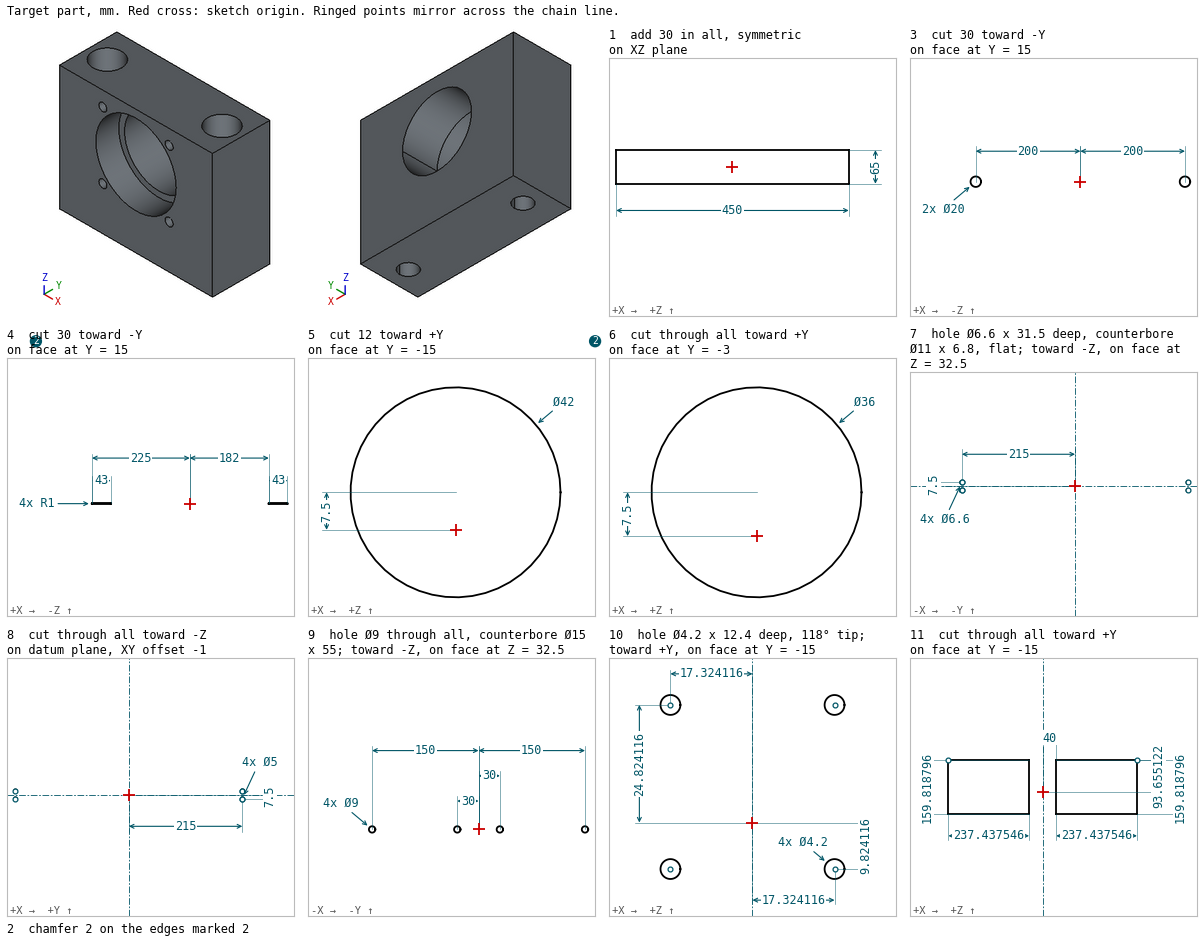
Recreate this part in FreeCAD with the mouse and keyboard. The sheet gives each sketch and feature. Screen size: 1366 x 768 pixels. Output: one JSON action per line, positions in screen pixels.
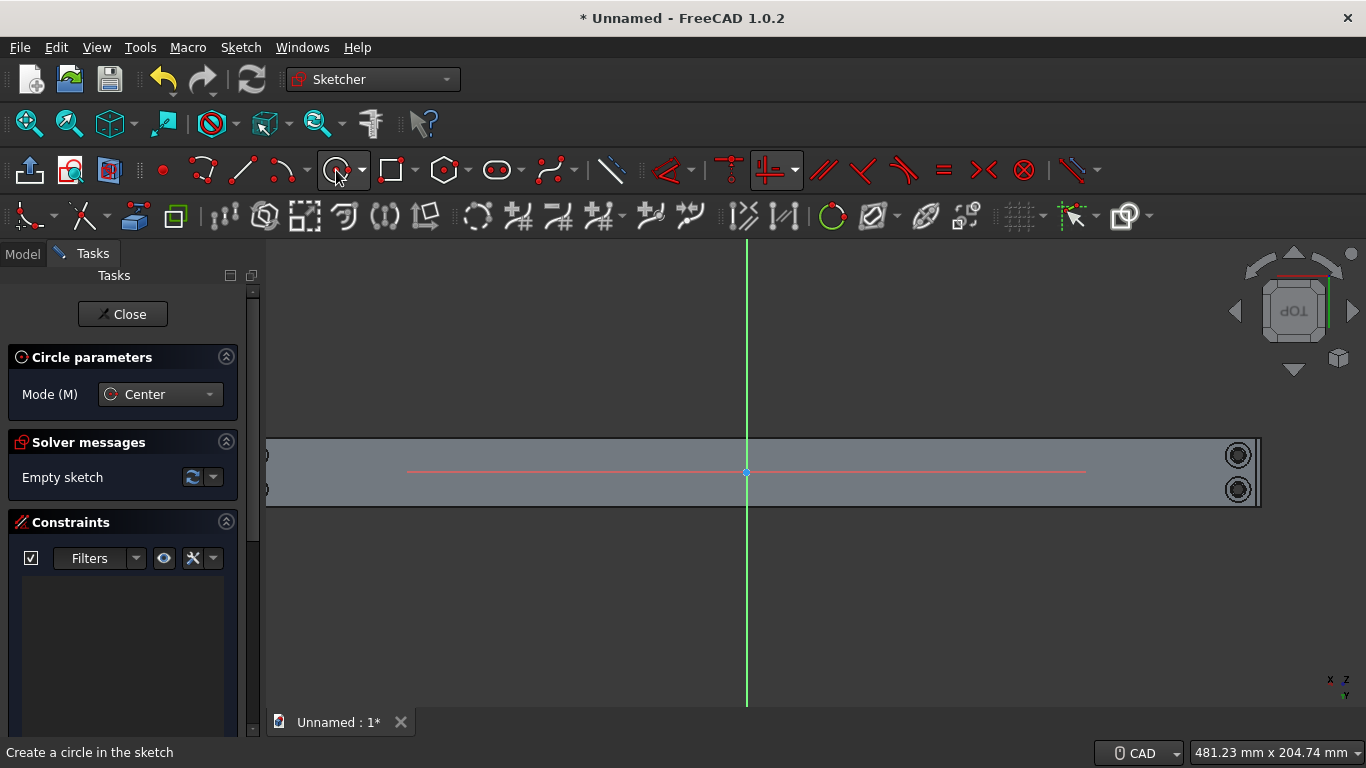
{"action": "scroll", "coordinate": [404, 472], "scroll_direction": "up", "scroll_amount": 4}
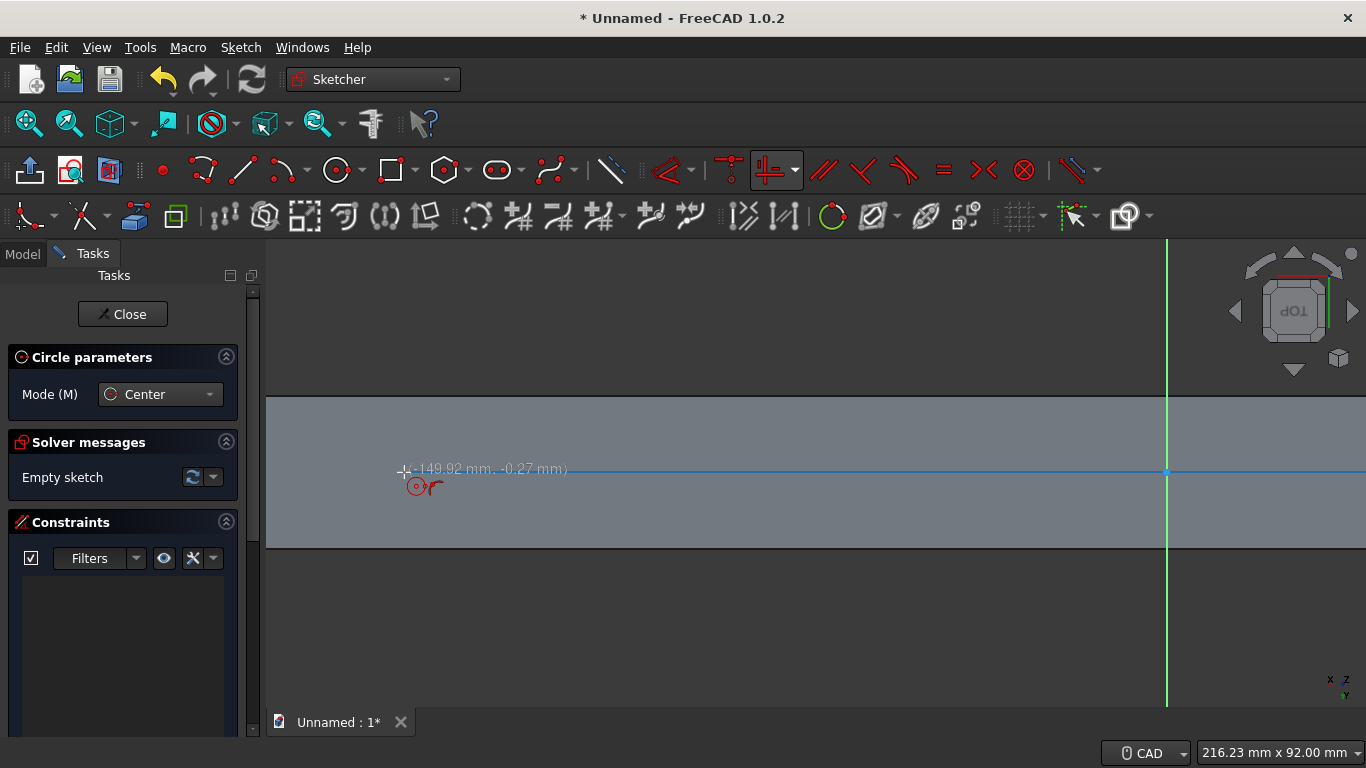
{"action": "left_click", "coordinate": [403, 472]}
{"action": "mouse_move", "coordinate": [420, 456]}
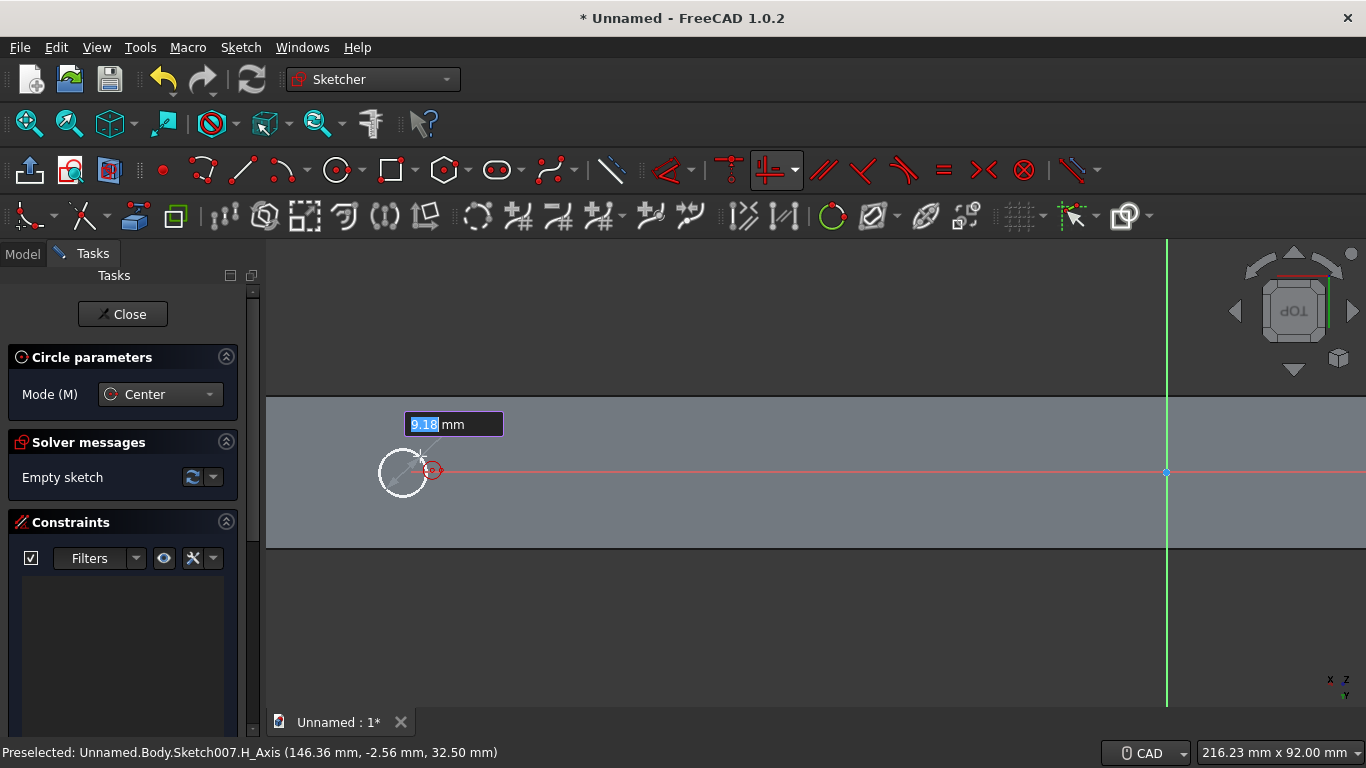
{"action": "type", "text": "9"}
{"action": "key", "text": "Return"}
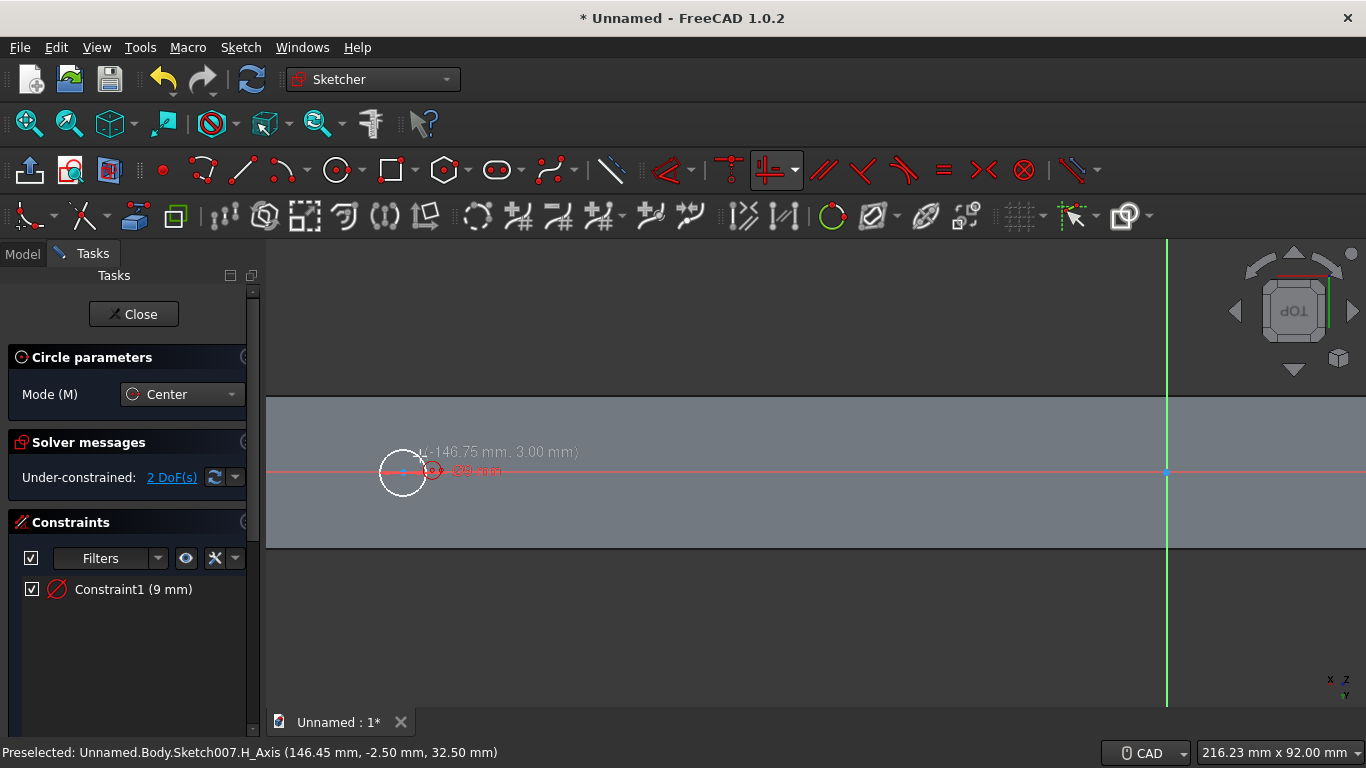
{"action": "left_click", "coordinate": [1014, 472]}
{"action": "mouse_move", "coordinate": [1030, 456]}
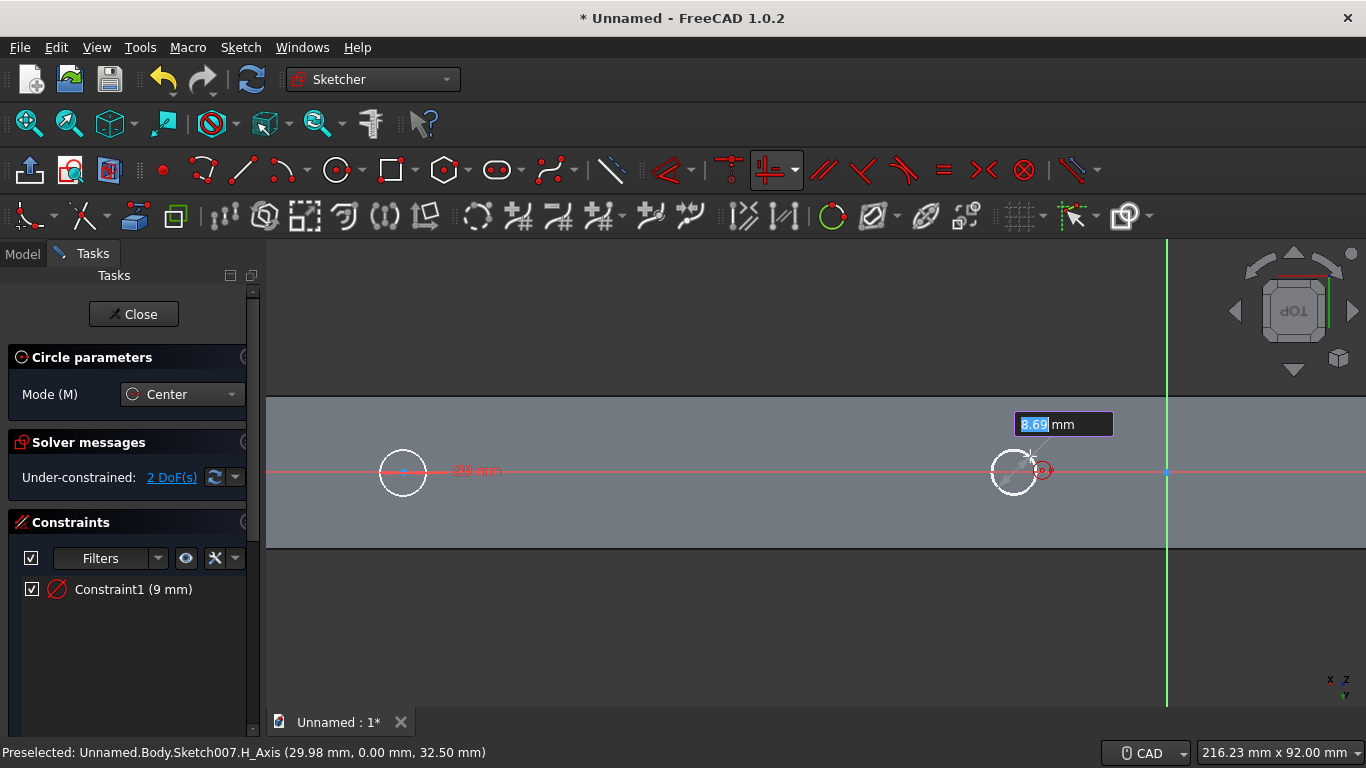
{"action": "type", "text": "9"}
{"action": "key", "text": "Return"}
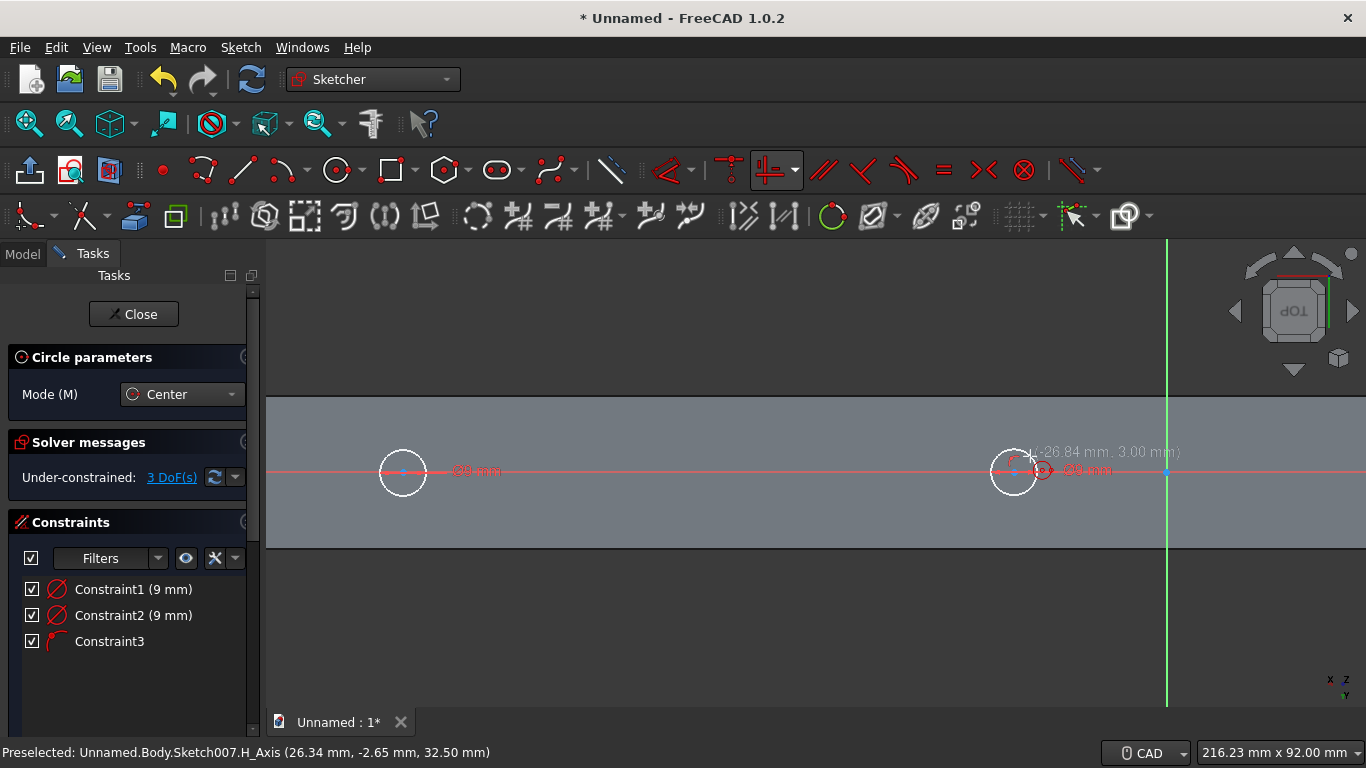
{"action": "scroll", "coordinate": [406, 474], "scroll_direction": "down", "scroll_amount": 4}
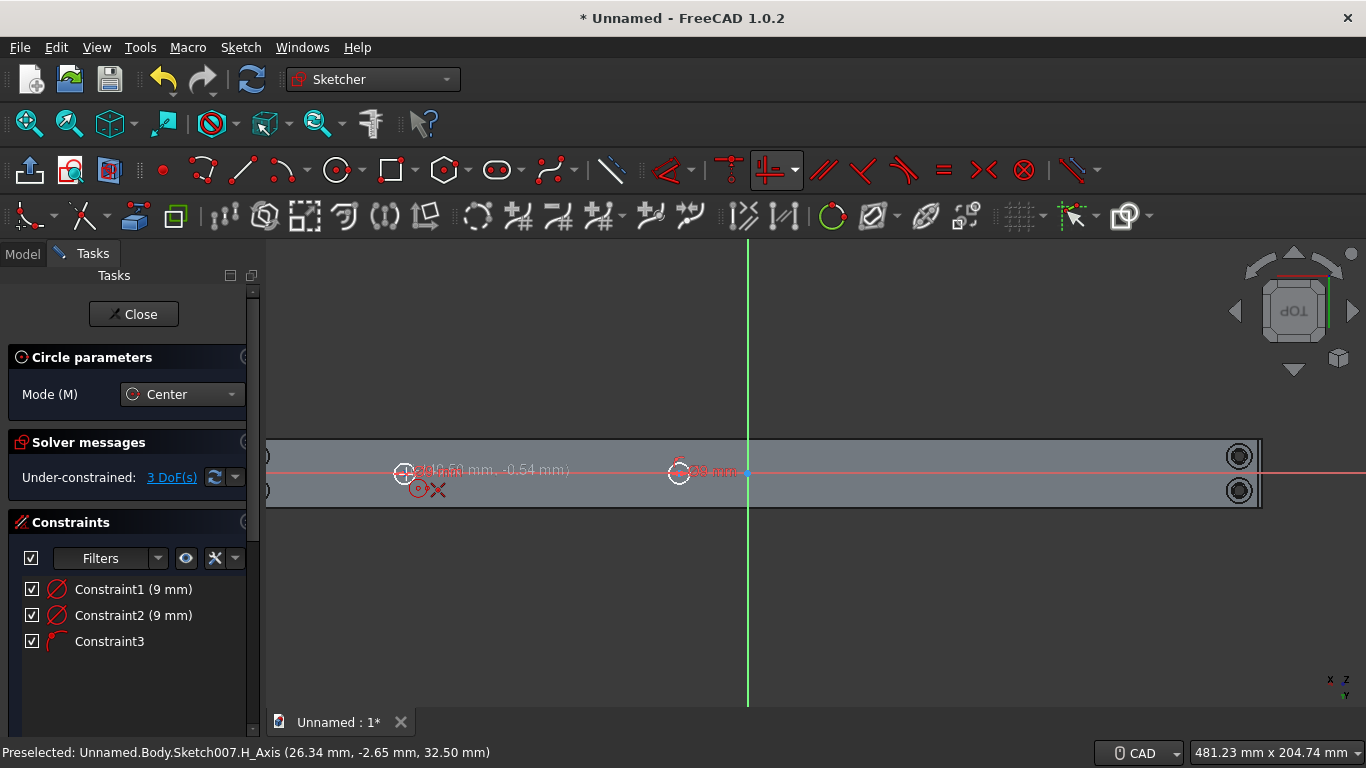
{"action": "scroll", "coordinate": [816, 473], "scroll_direction": "up", "scroll_amount": 4}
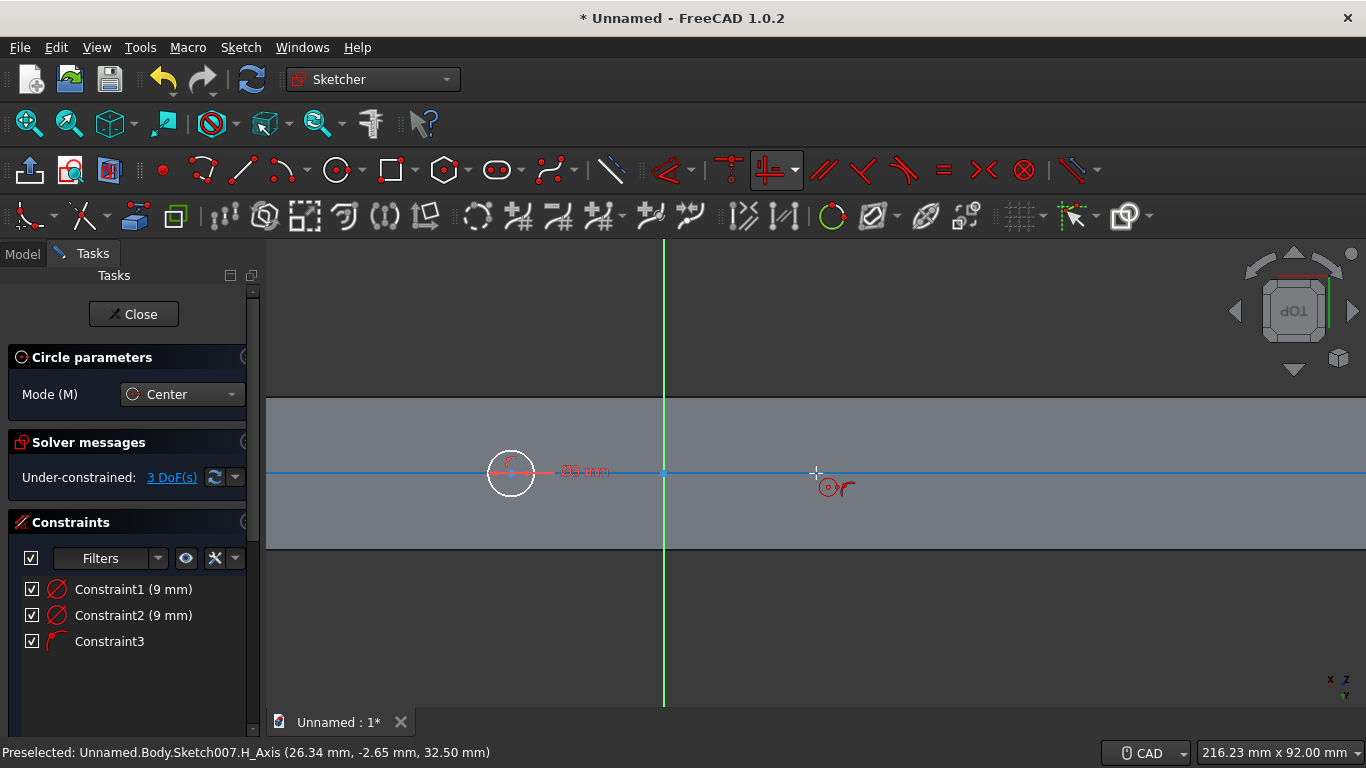
{"action": "left_click", "coordinate": [816, 473]}
{"action": "mouse_move", "coordinate": [832, 457]}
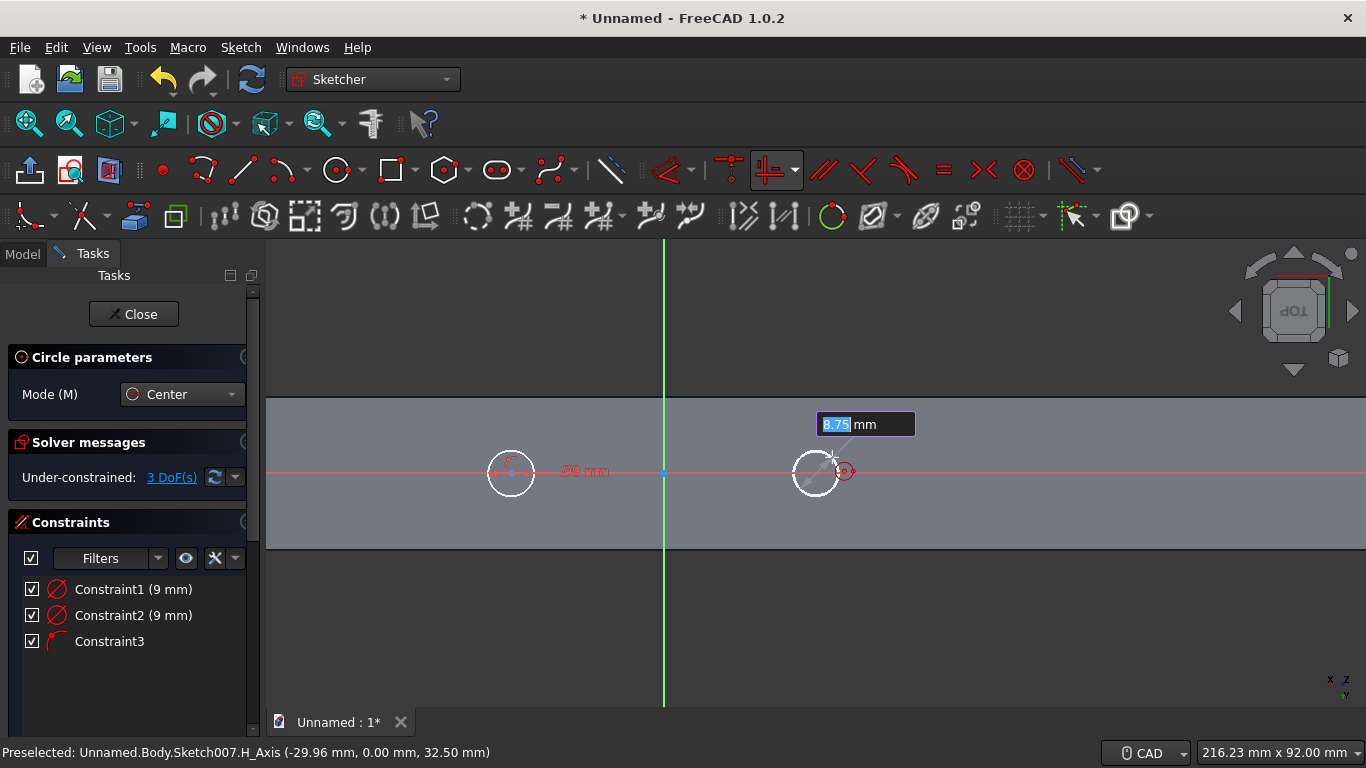
{"action": "type", "text": "9"}
{"action": "key", "text": "Return"}